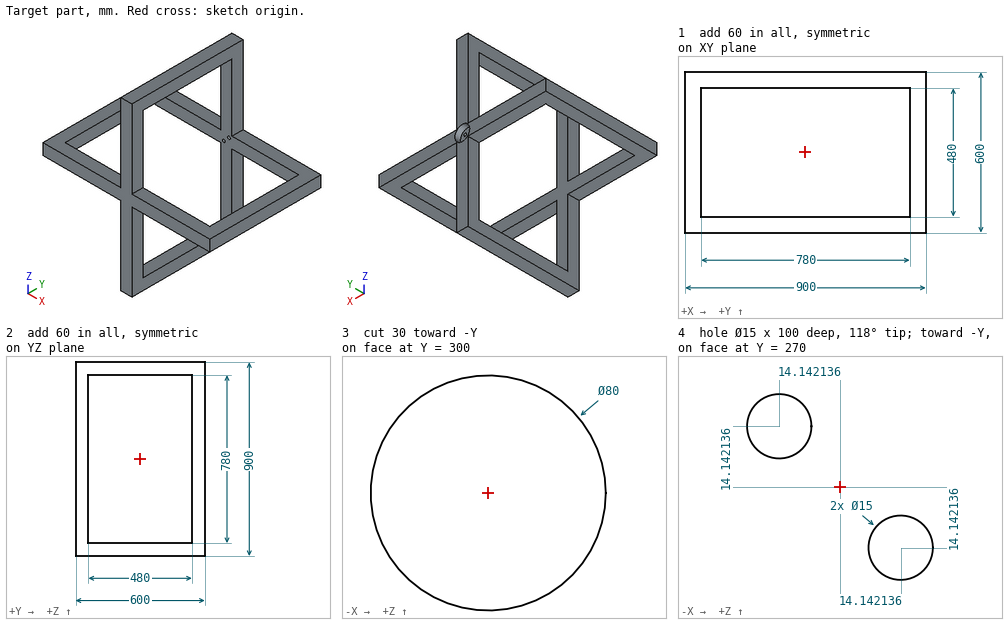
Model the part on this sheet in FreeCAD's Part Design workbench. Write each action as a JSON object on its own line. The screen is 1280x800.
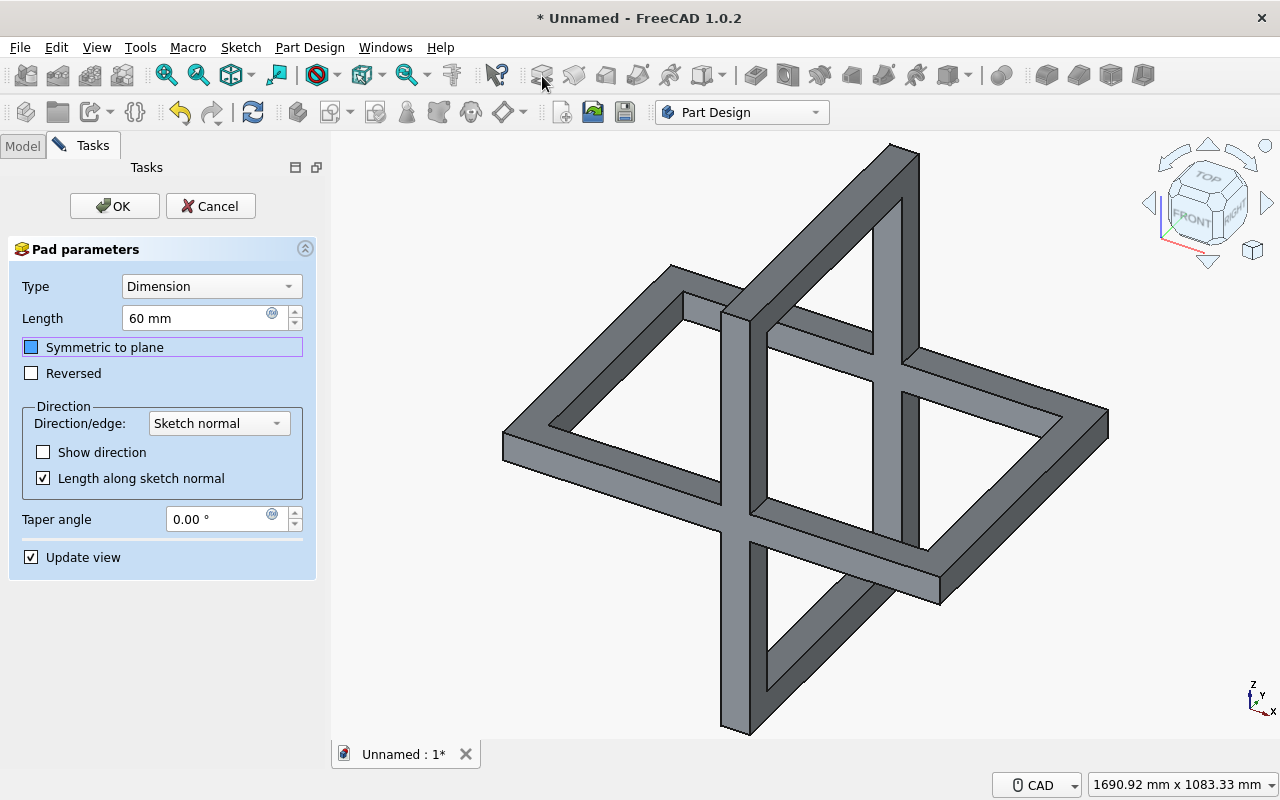
{"action": "left_click", "coordinate": [30, 347]}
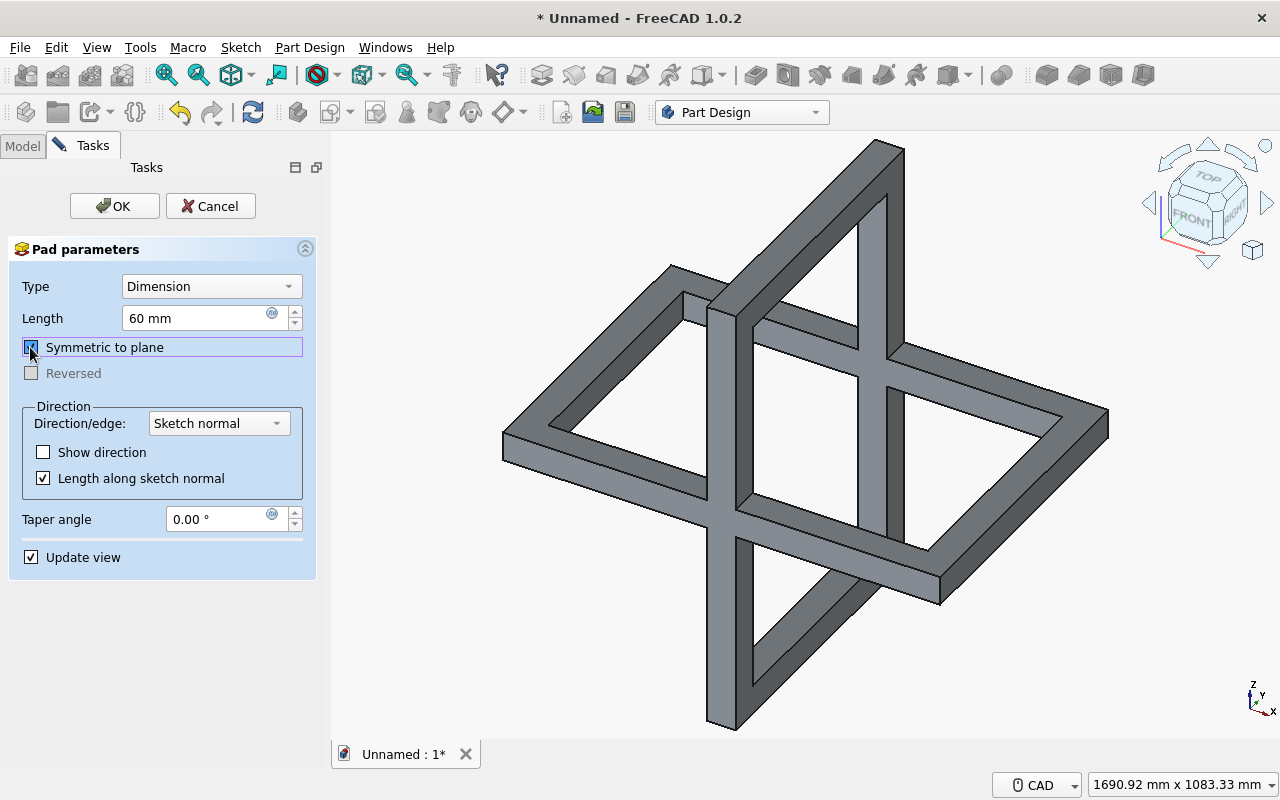
{"action": "left_click", "coordinate": [115, 206]}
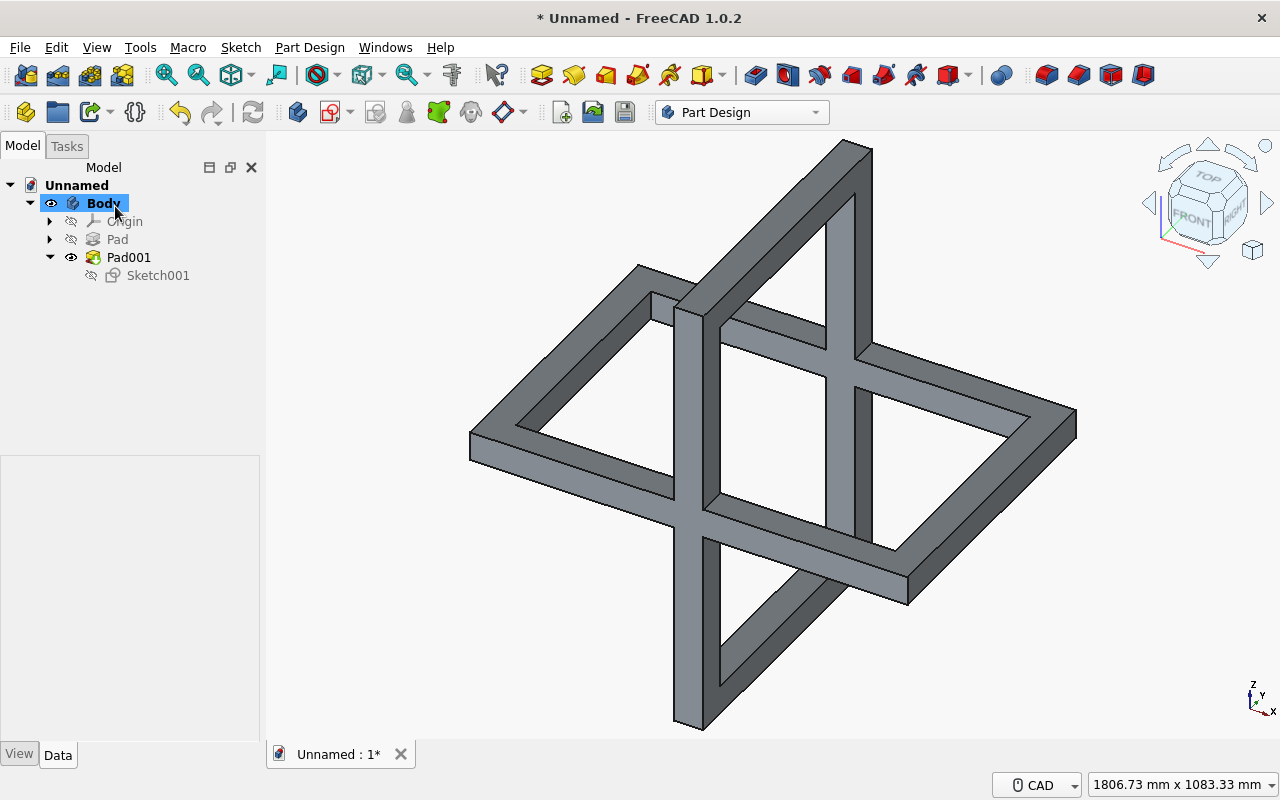
{"action": "left_click", "coordinate": [168, 76]}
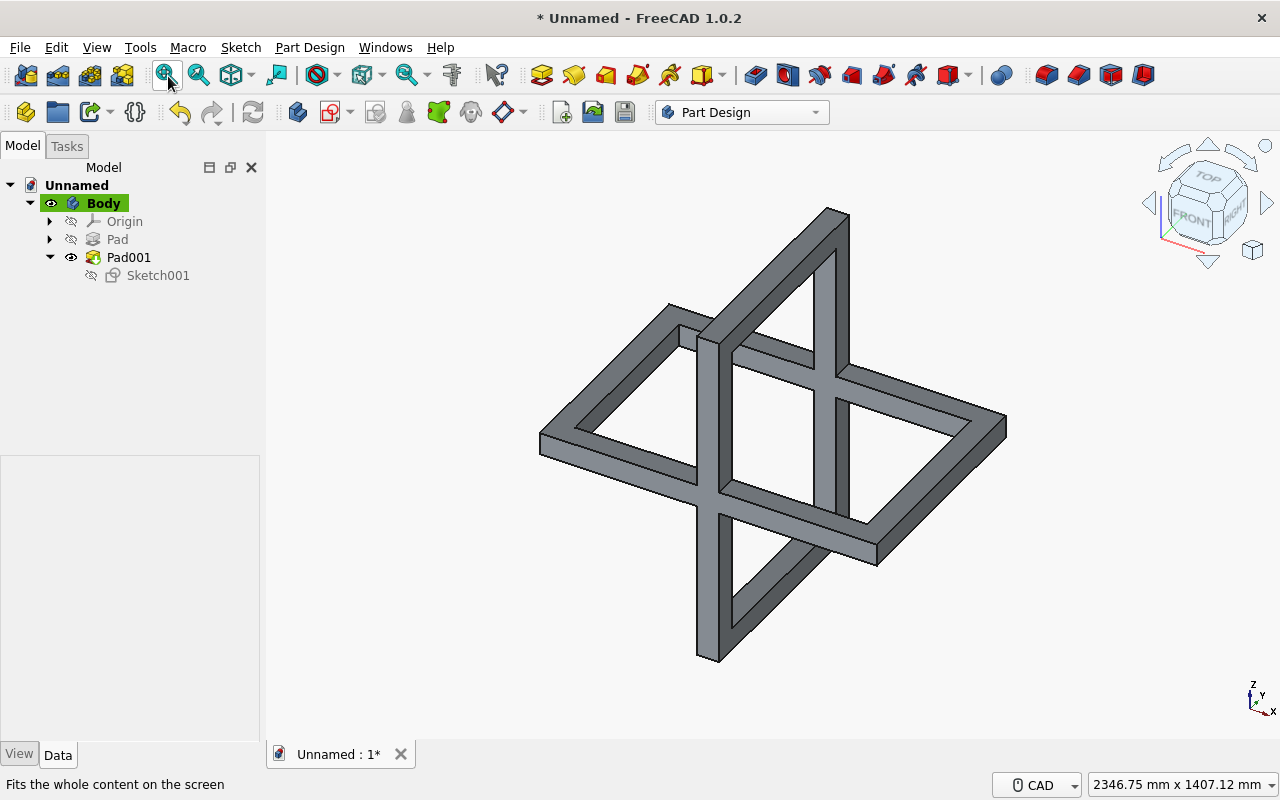
{"action": "key", "text": "4"}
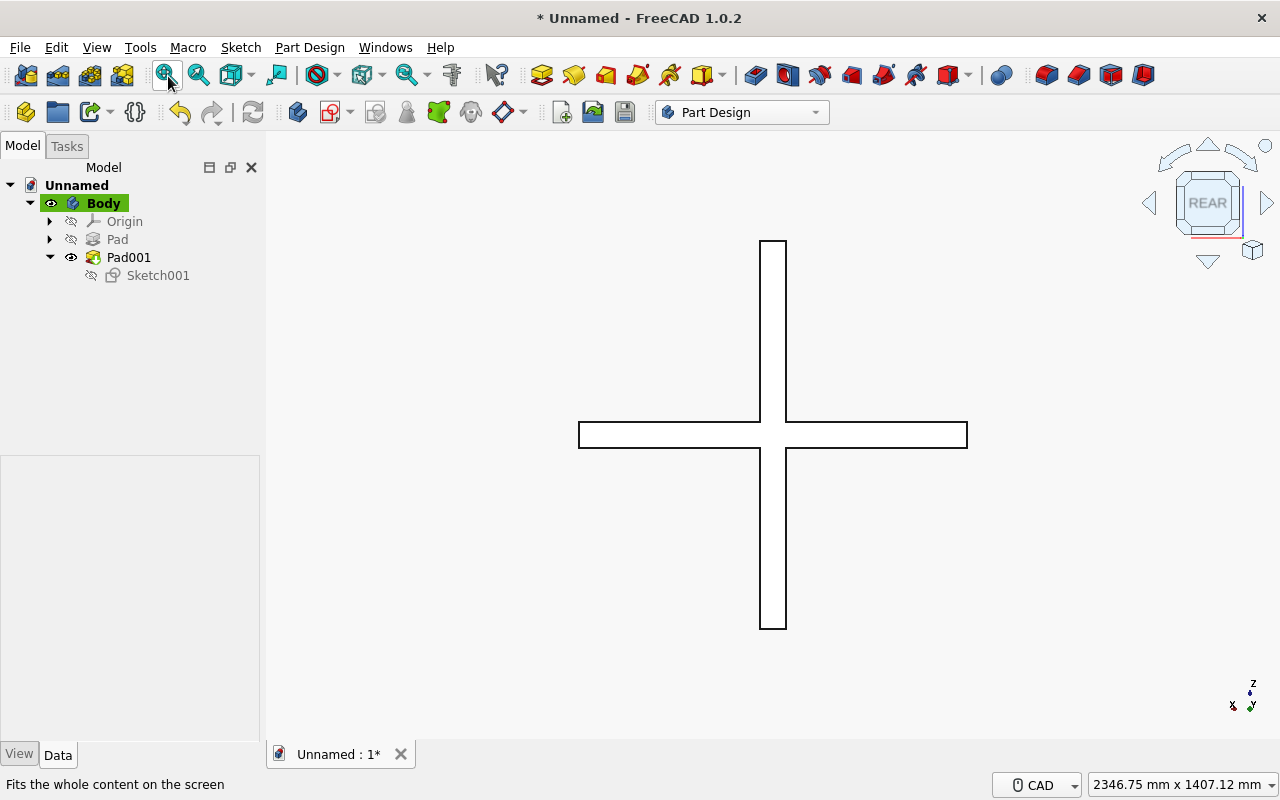
{"action": "left_click", "coordinate": [773, 434]}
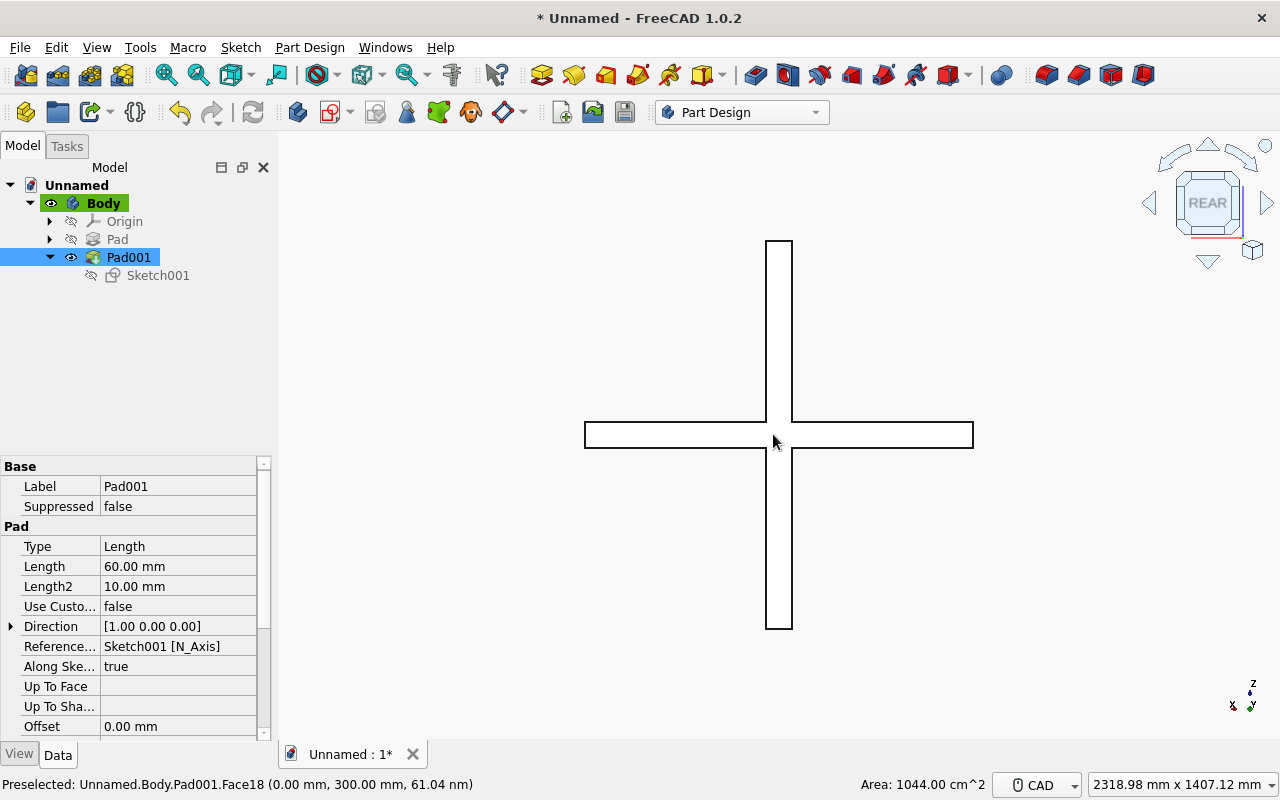
{"action": "left_click", "coordinate": [330, 112]}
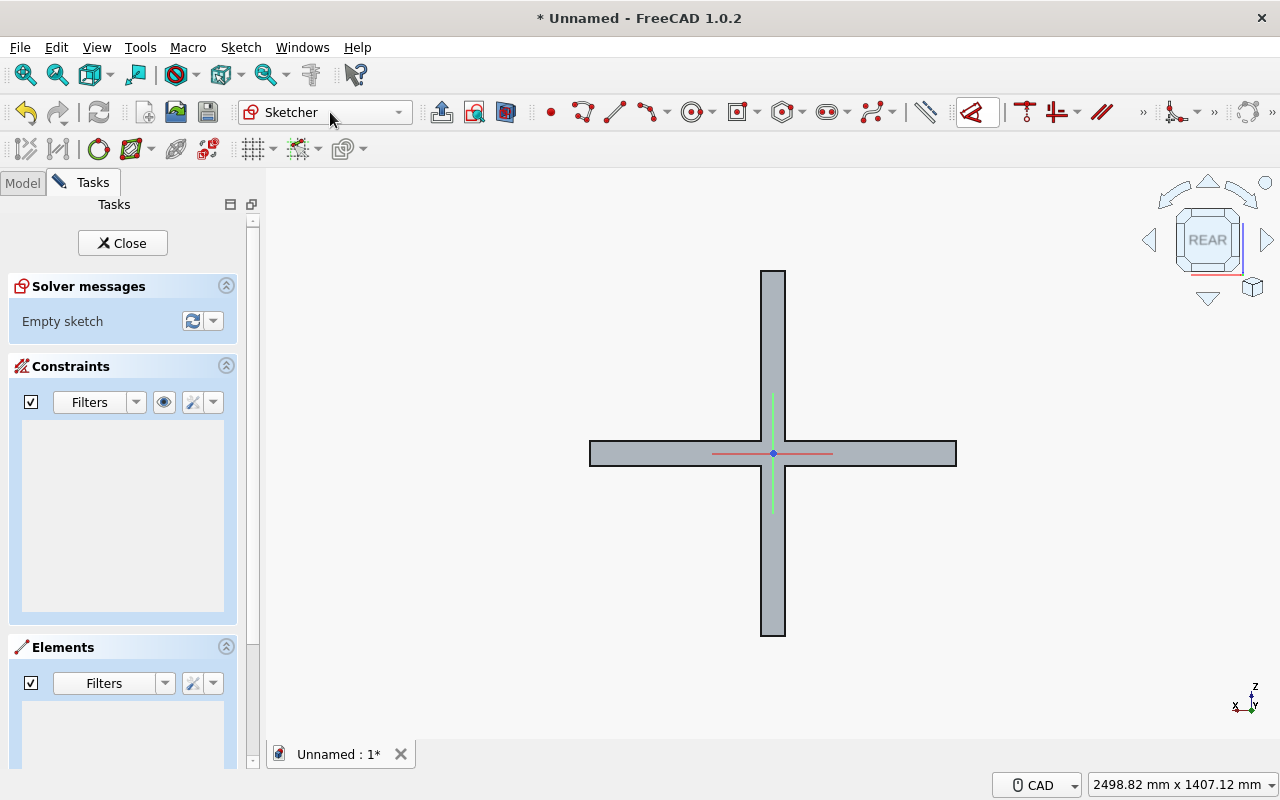
{"action": "scroll", "coordinate": [780, 454], "scroll_direction": "up", "scroll_amount": 12}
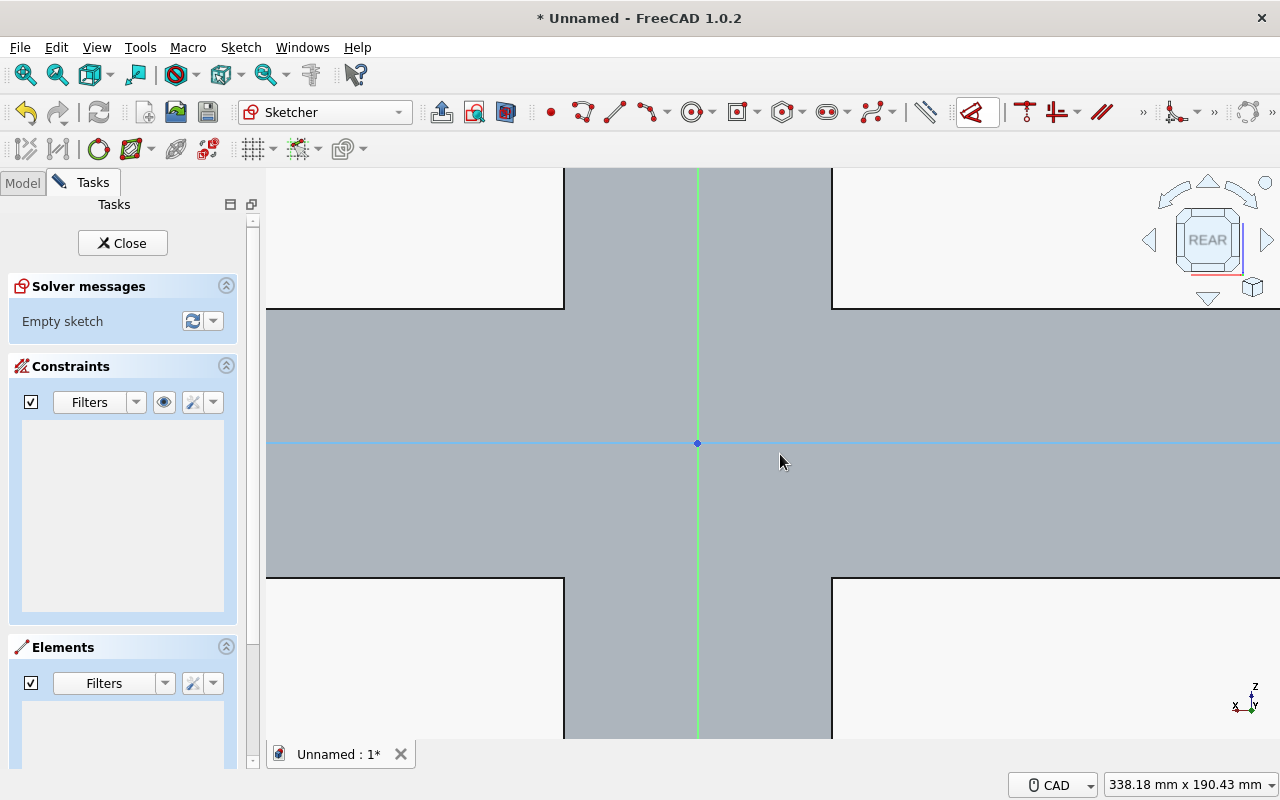
{"action": "left_click", "coordinate": [692, 112]}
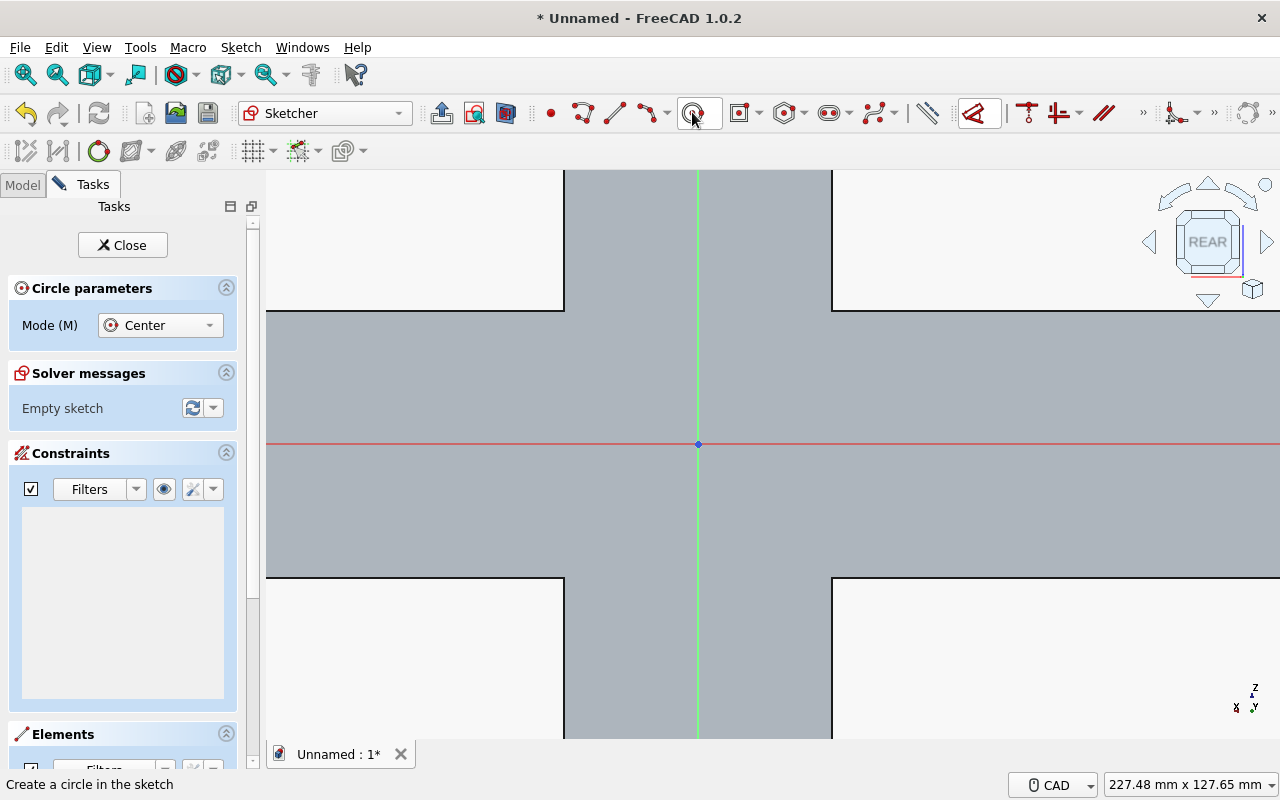
{"action": "left_click", "coordinate": [698, 444]}
{"action": "mouse_move", "coordinate": [824, 318]}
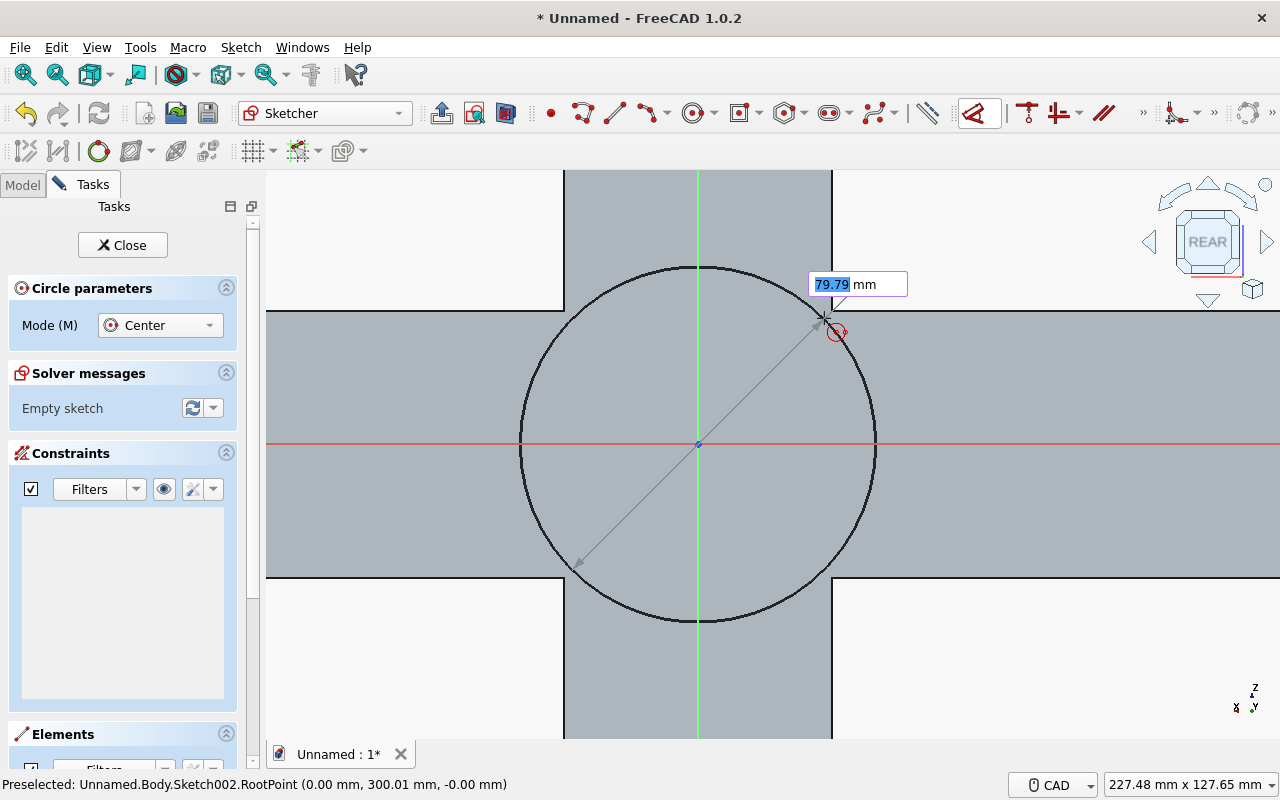
{"action": "type", "text": "80"}
{"action": "key", "text": "Return"}
{"action": "key", "text": "Escape"}